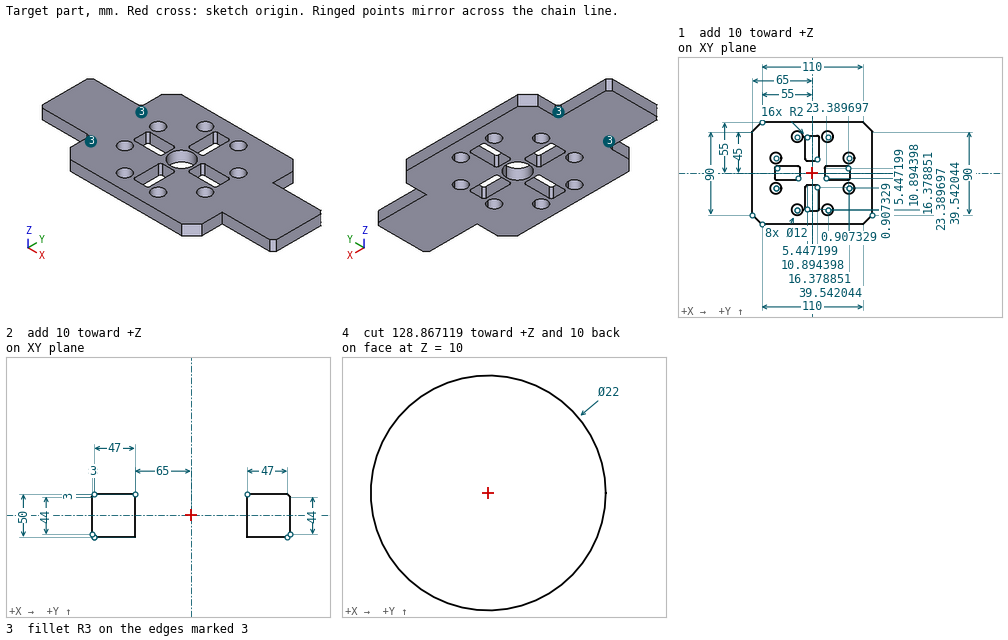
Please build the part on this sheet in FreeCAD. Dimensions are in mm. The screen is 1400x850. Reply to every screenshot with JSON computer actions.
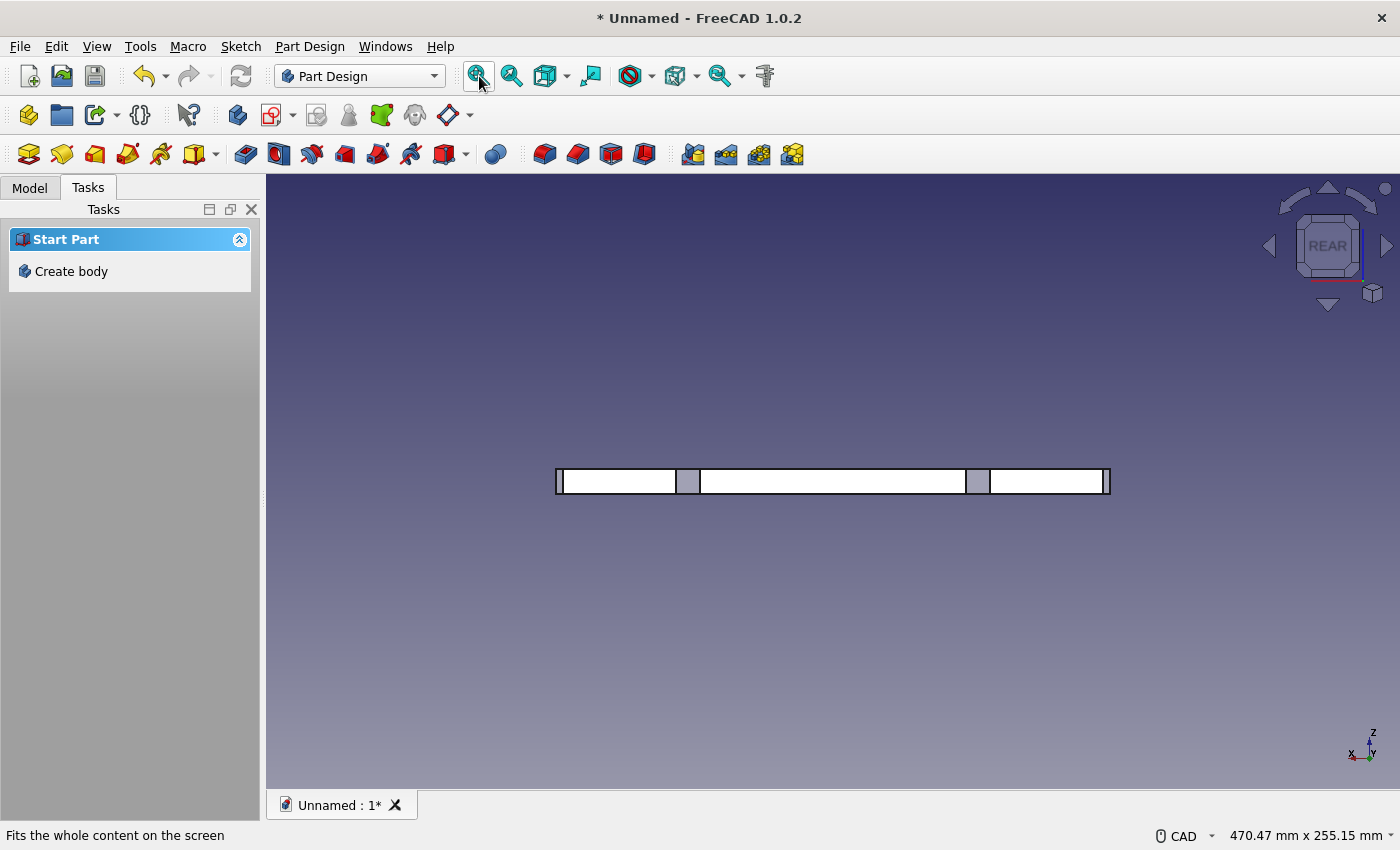
{"action": "key", "text": "6"}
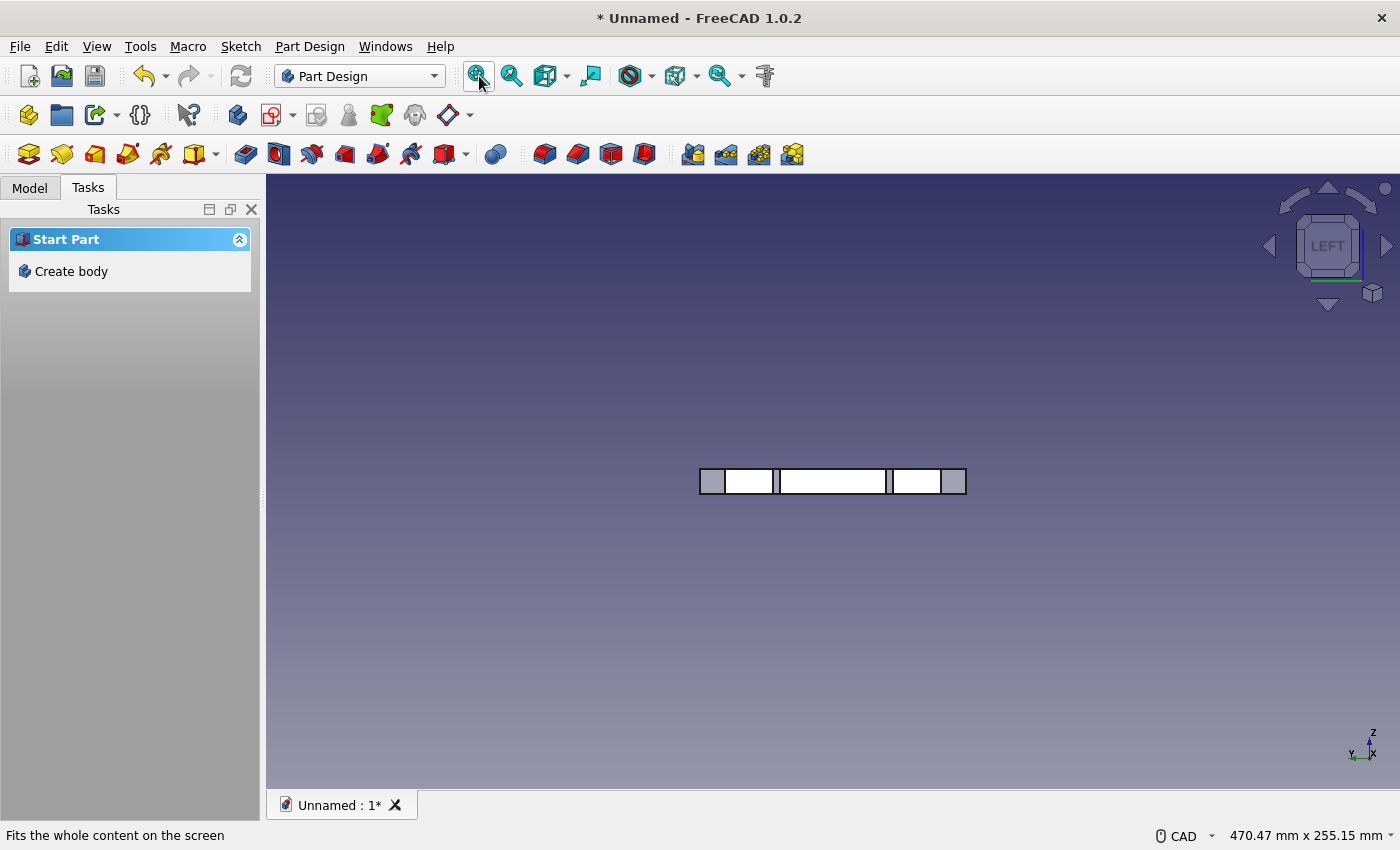
{"action": "left_click", "coordinate": [479, 76]}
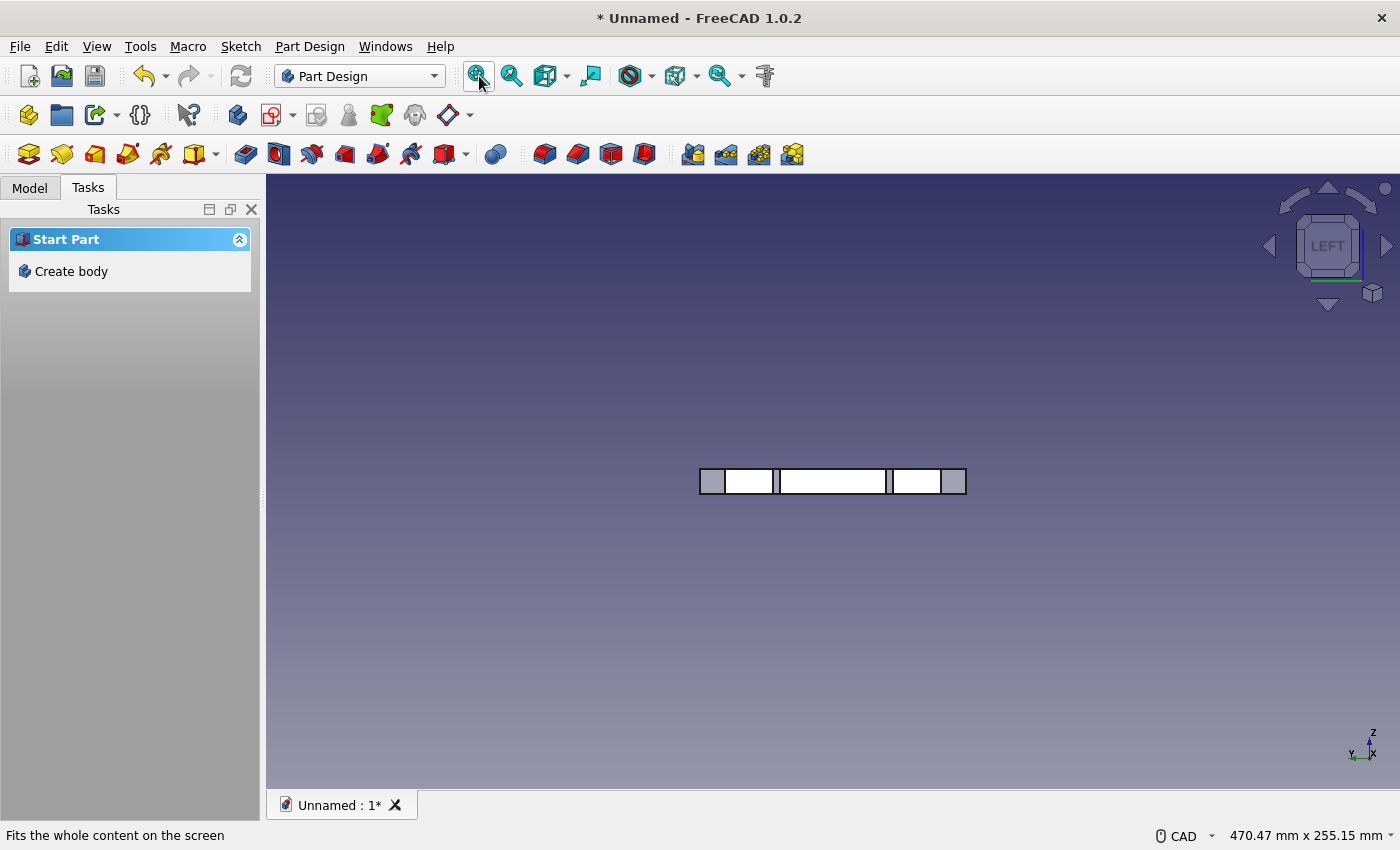
{"action": "key", "text": "v 3"}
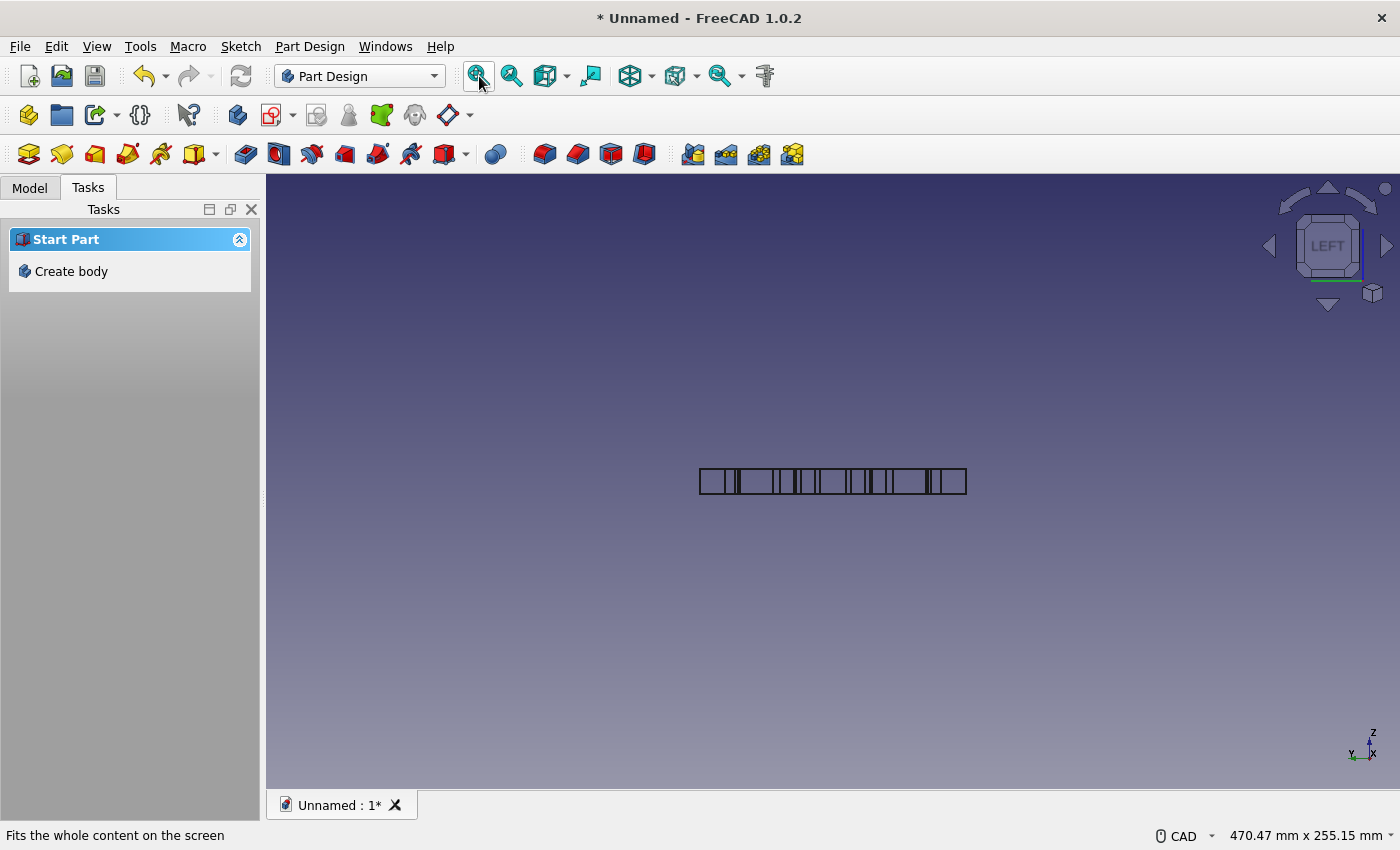
{"action": "key", "text": "0"}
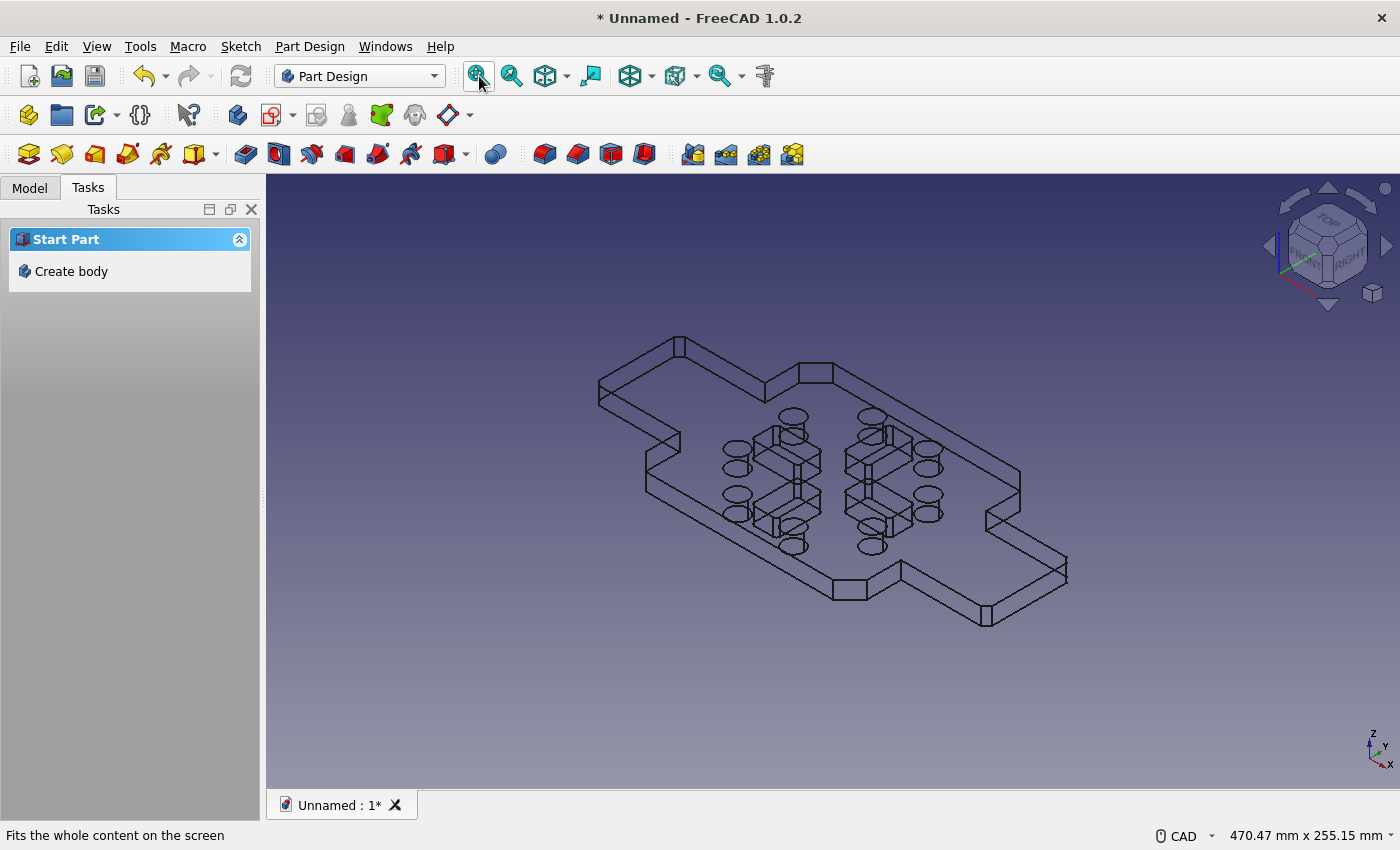
{"action": "left_click", "coordinate": [765, 392]}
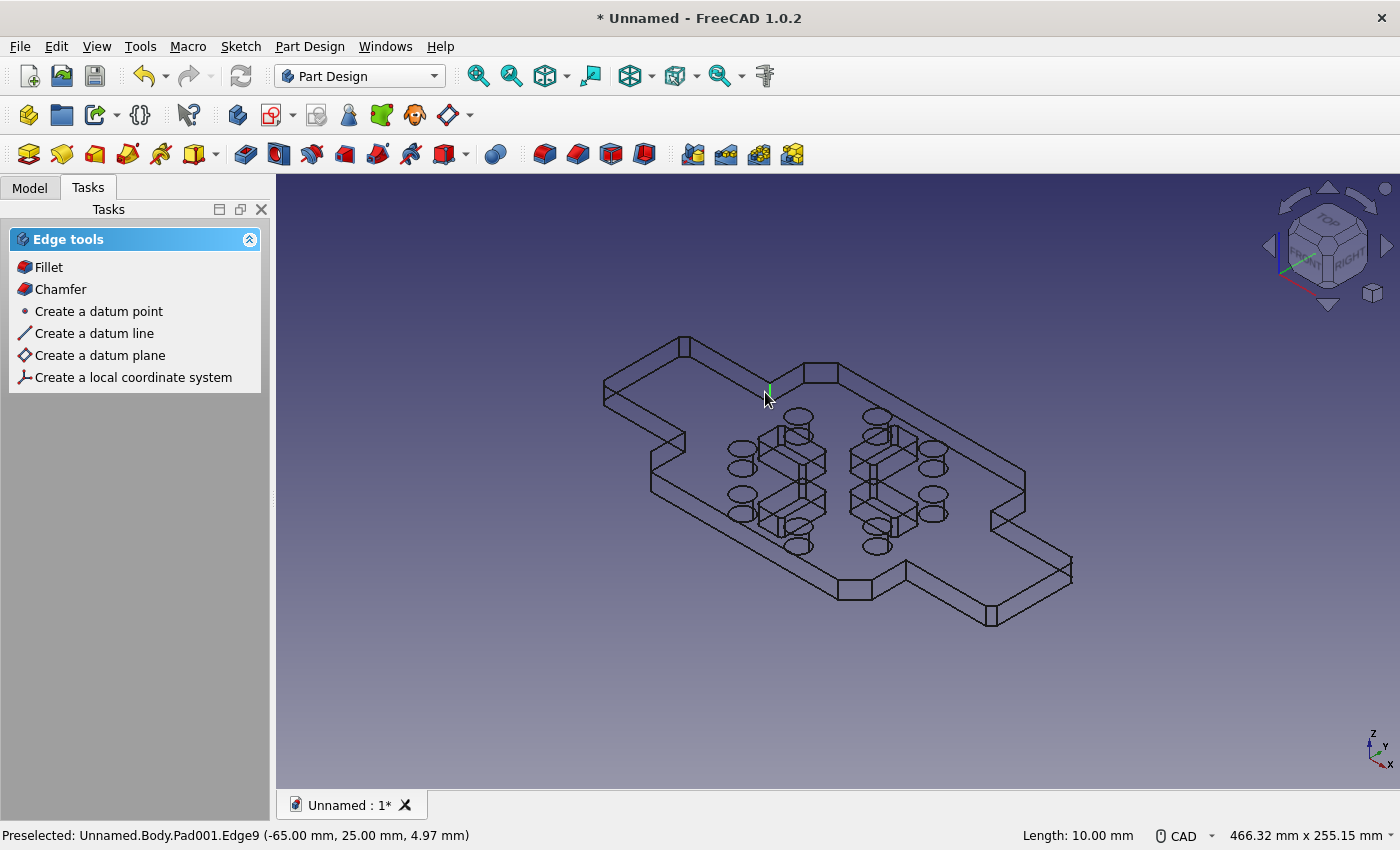
{"action": "left_click", "coordinate": [685, 441], "text": "ctrl"}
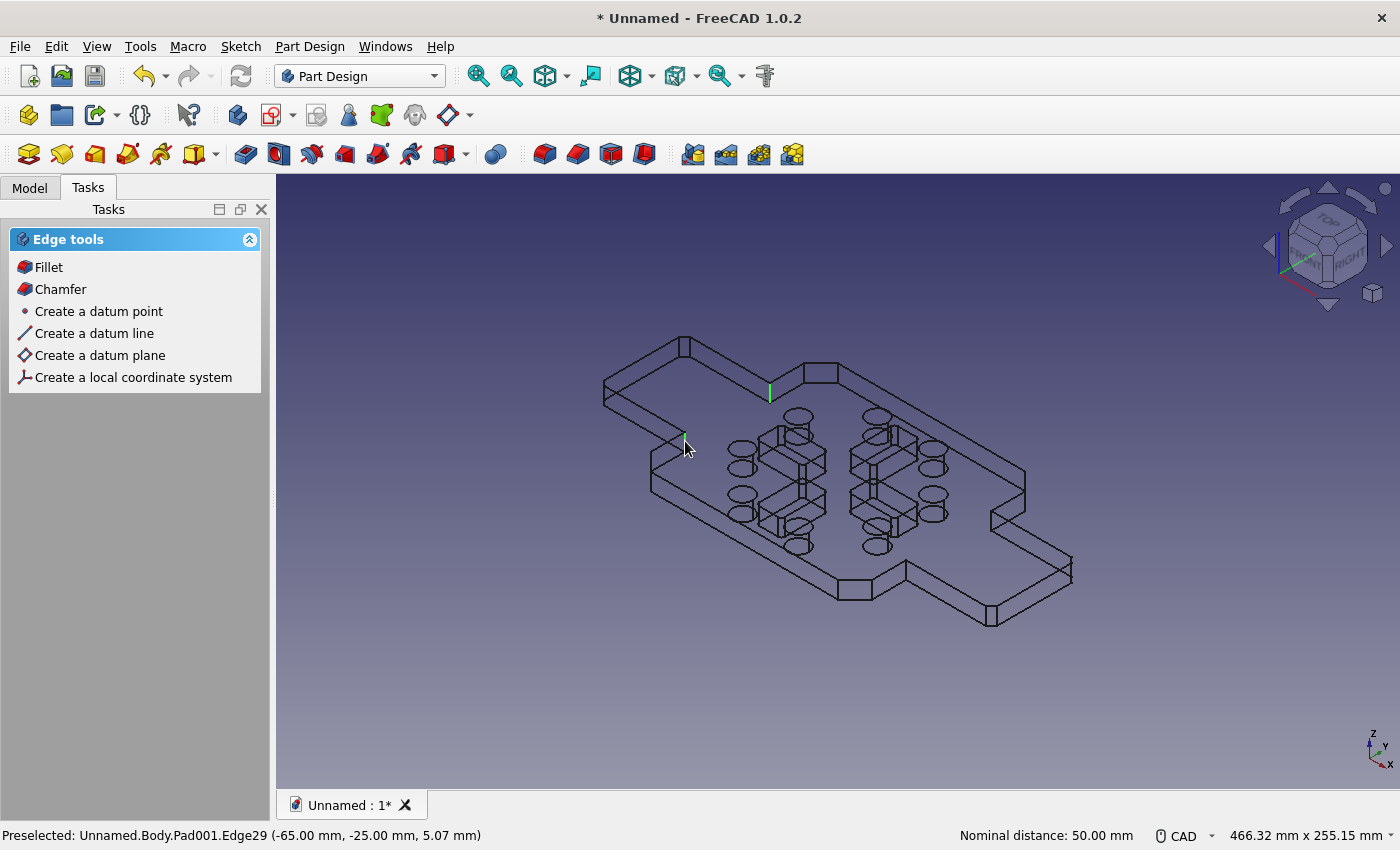
{"action": "key", "text": "v 1"}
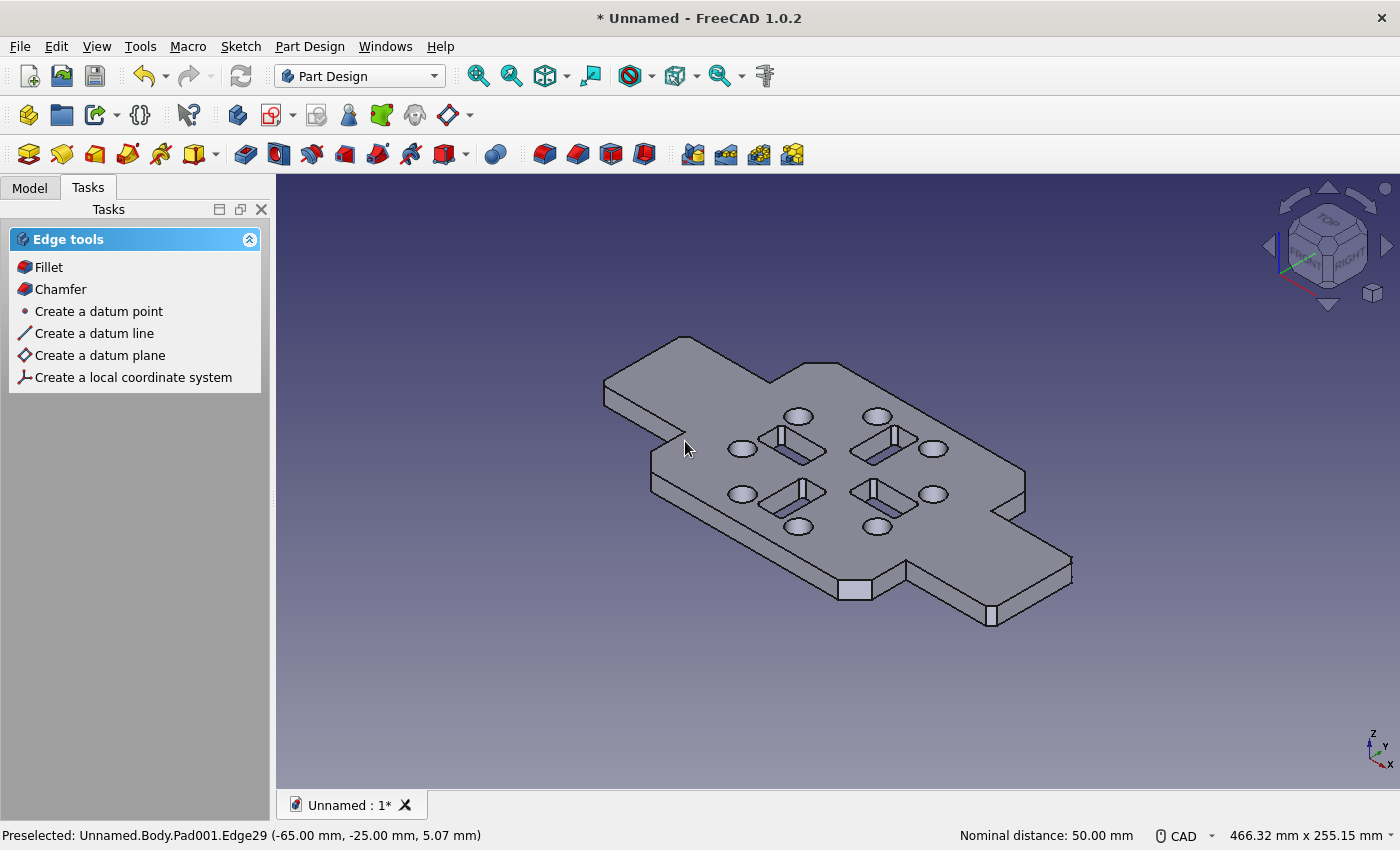
{"action": "left_click", "coordinate": [545, 154]}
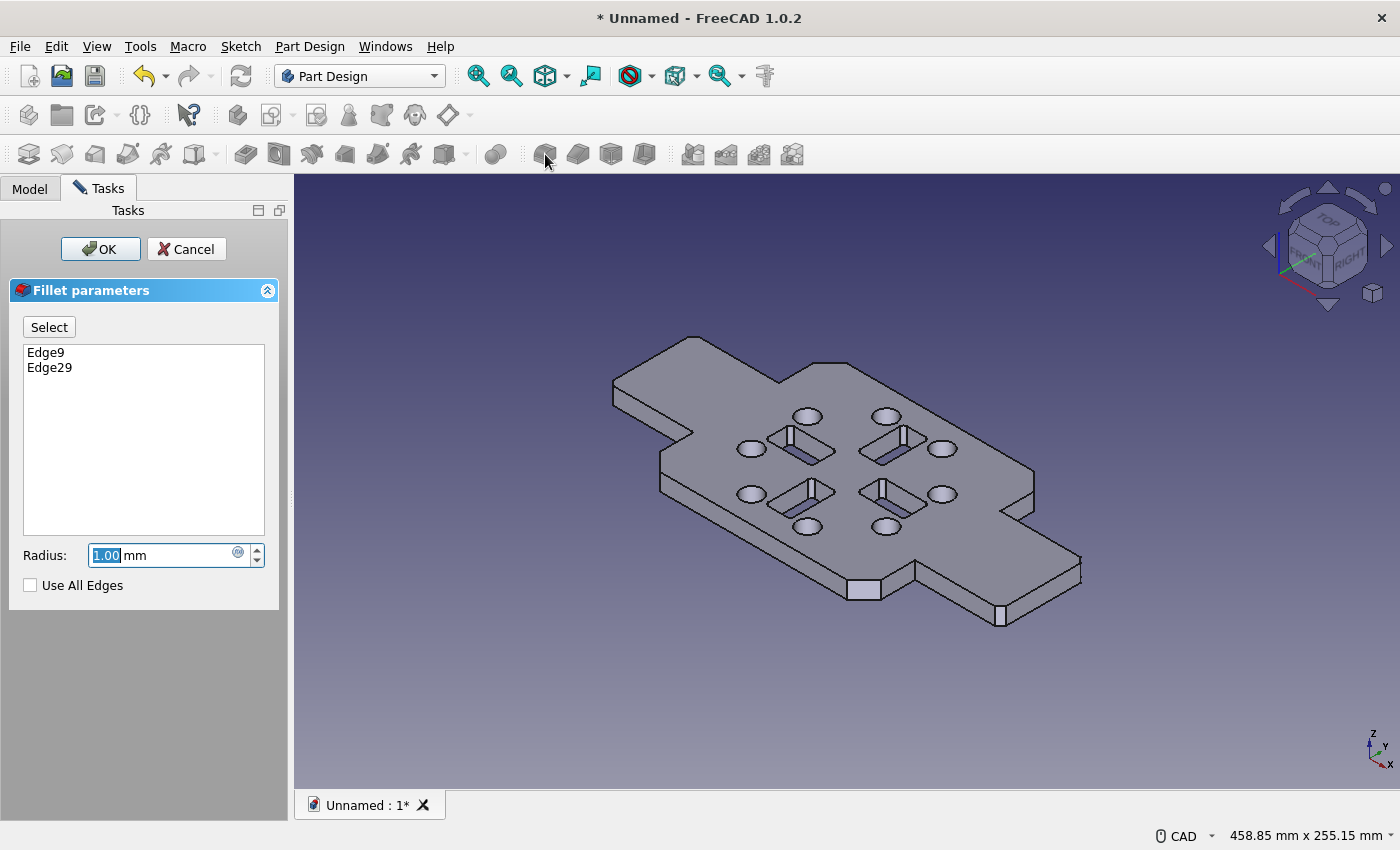
{"action": "type", "text": "3"}
{"action": "key", "text": "Tab"}